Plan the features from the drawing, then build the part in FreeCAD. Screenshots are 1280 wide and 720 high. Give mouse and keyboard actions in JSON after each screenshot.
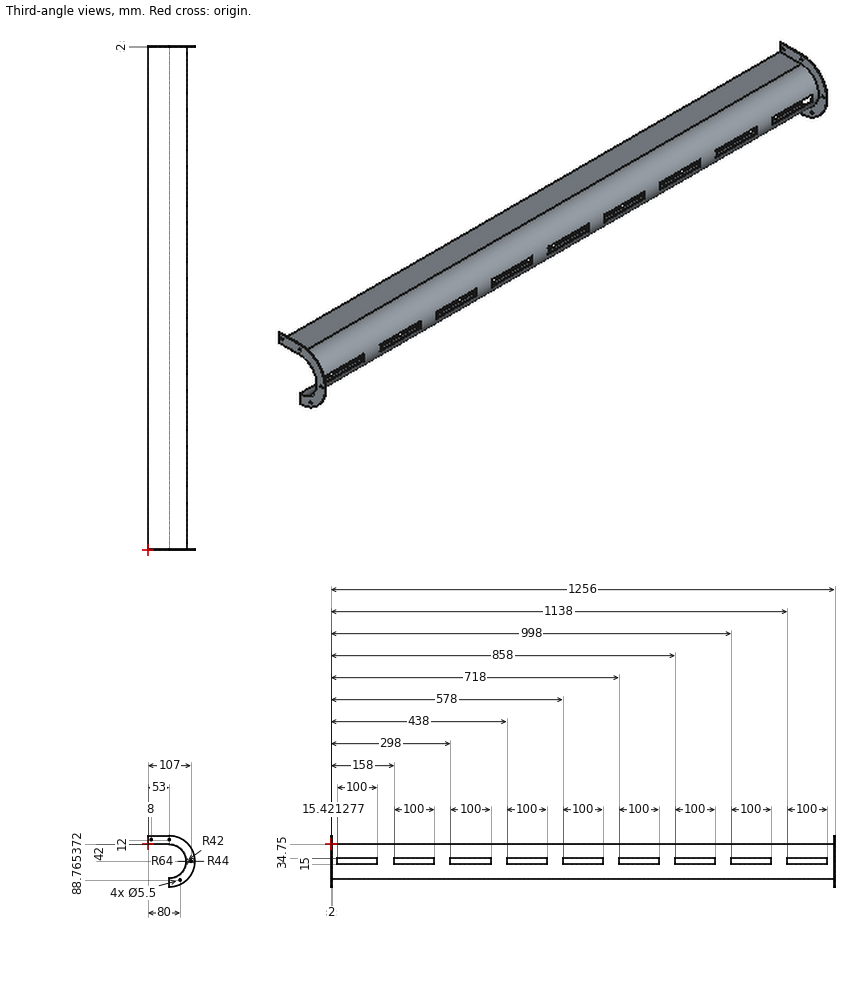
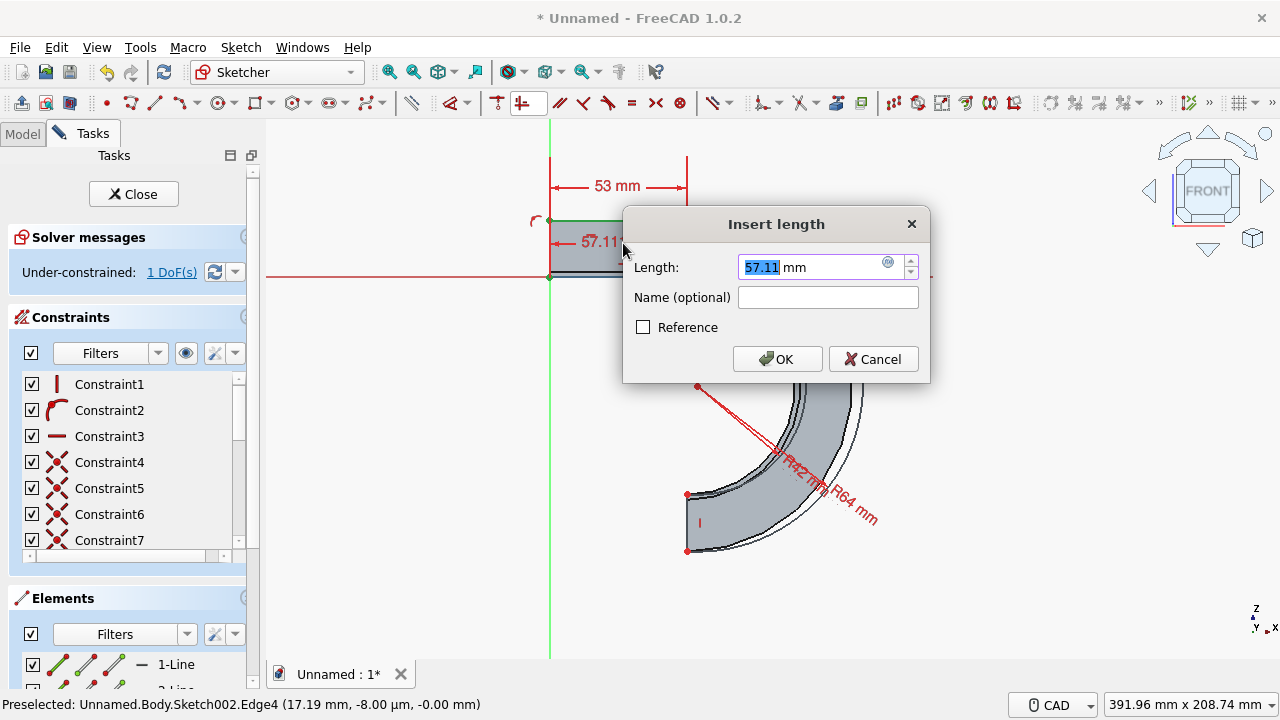
{"action": "type", "text": "53"}
{"action": "key", "text": "Return"}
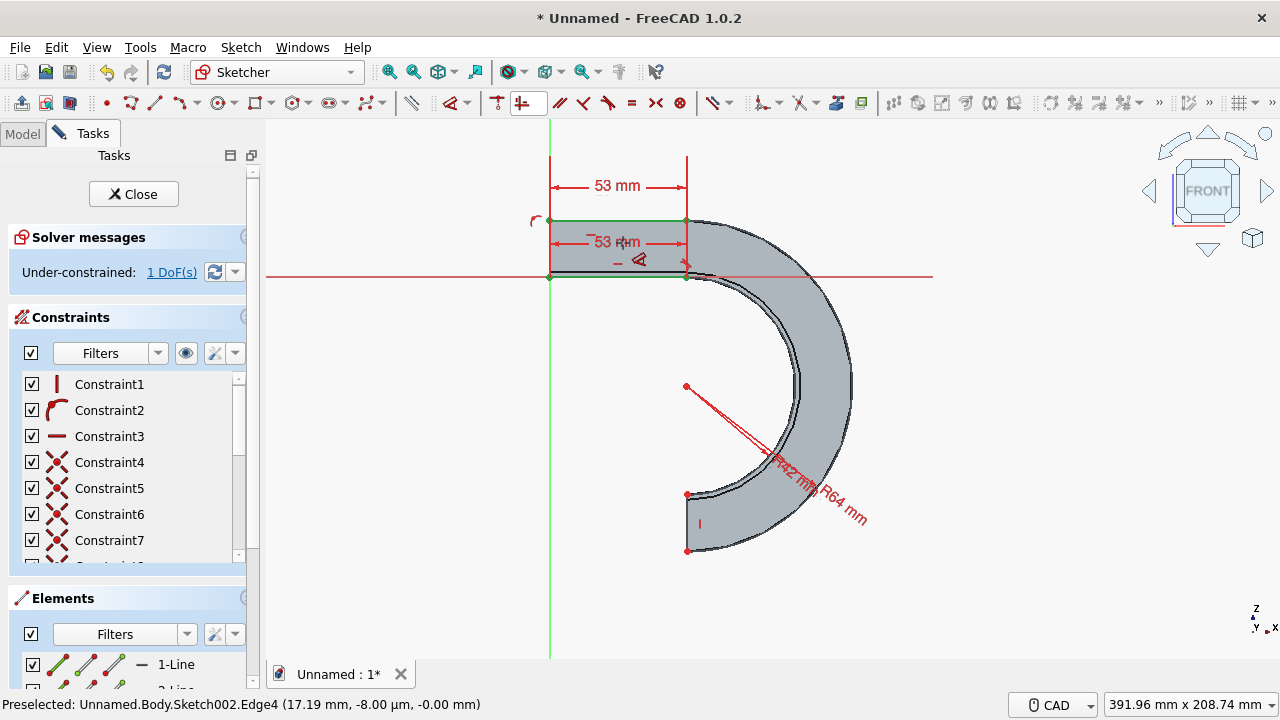
{"action": "left_click", "coordinate": [687, 495]}
{"action": "left_click", "coordinate": [618, 529]}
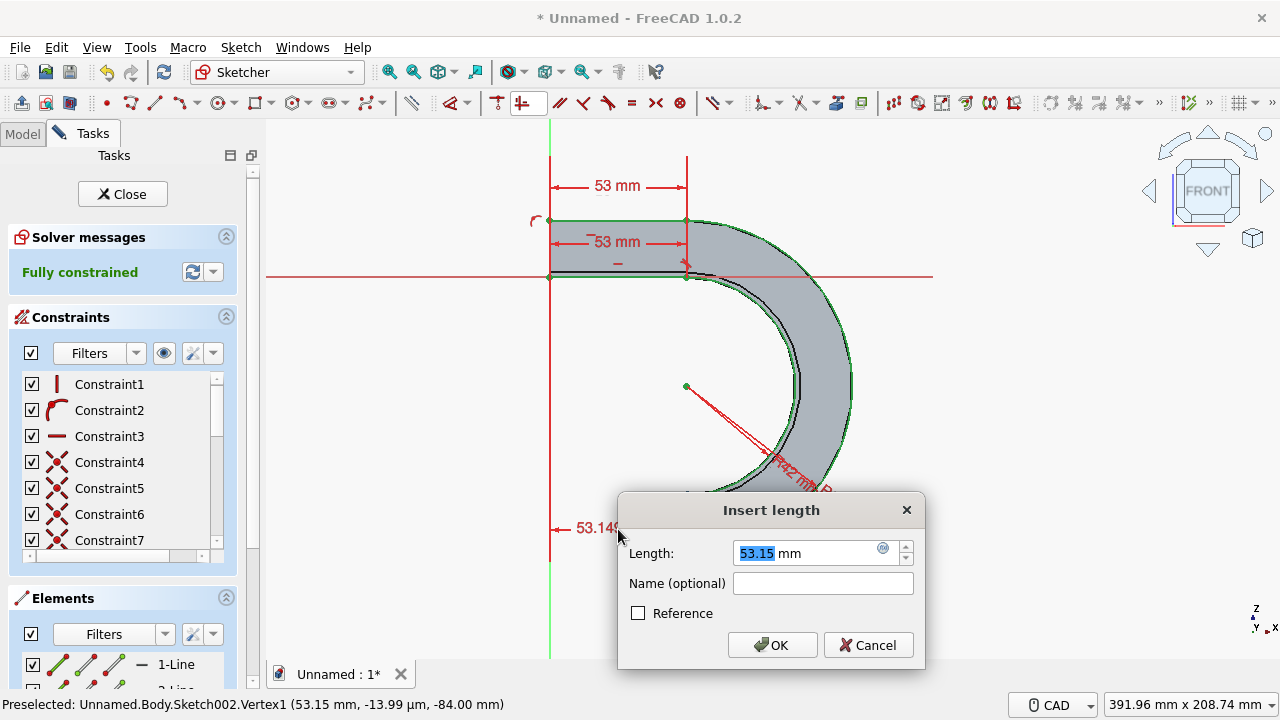
{"action": "type", "text": "53"}
{"action": "key", "text": "Return"}
{"action": "key", "text": "Escape"}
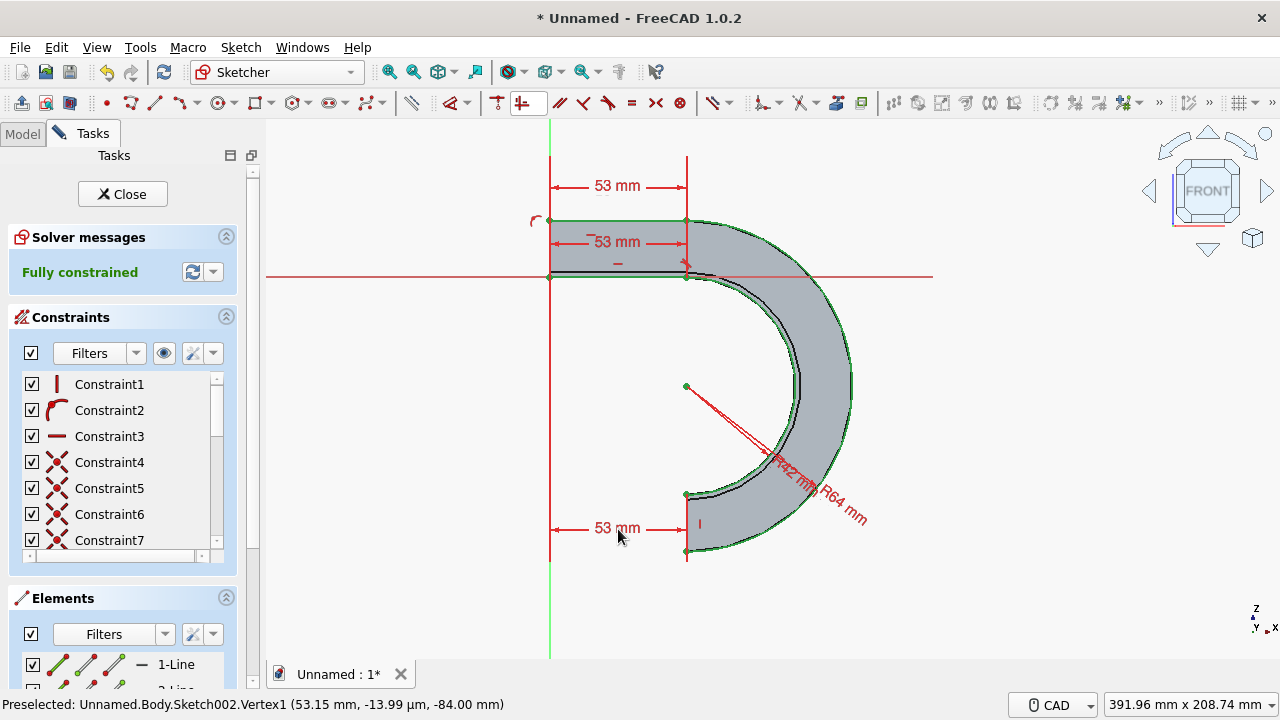
{"action": "left_click", "coordinate": [123, 194]}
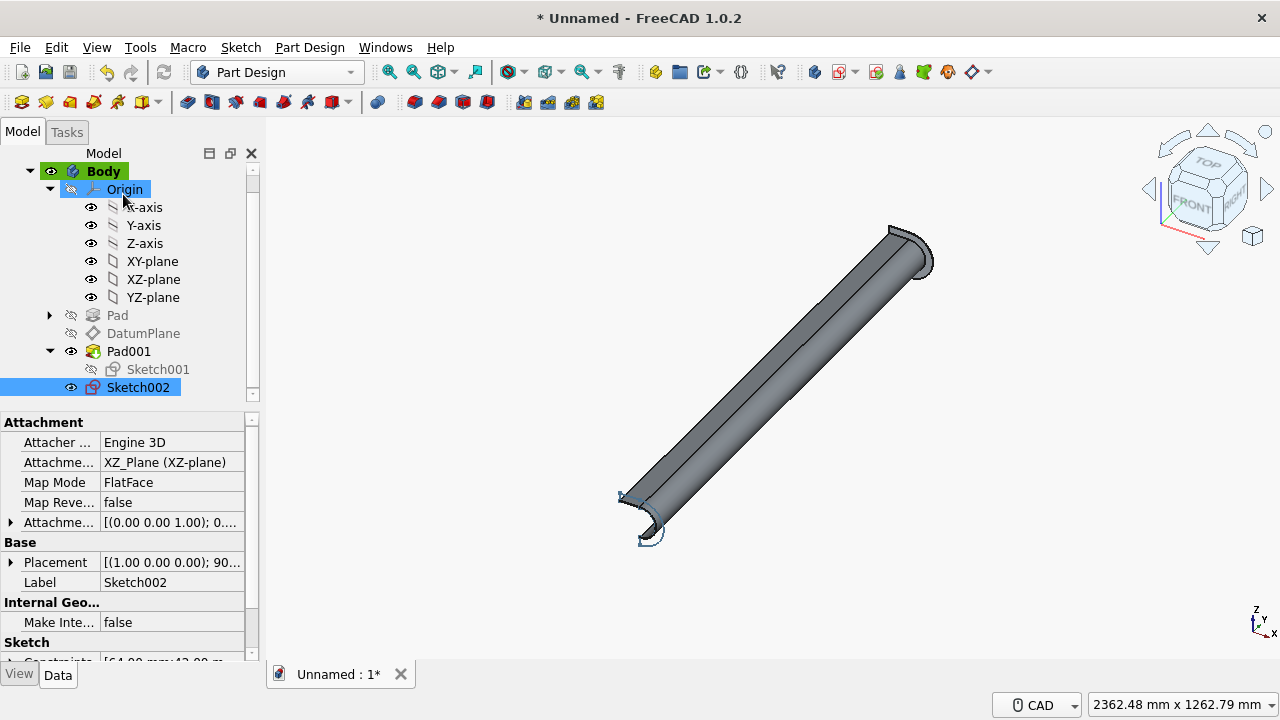
{"action": "left_click", "coordinate": [22, 102]}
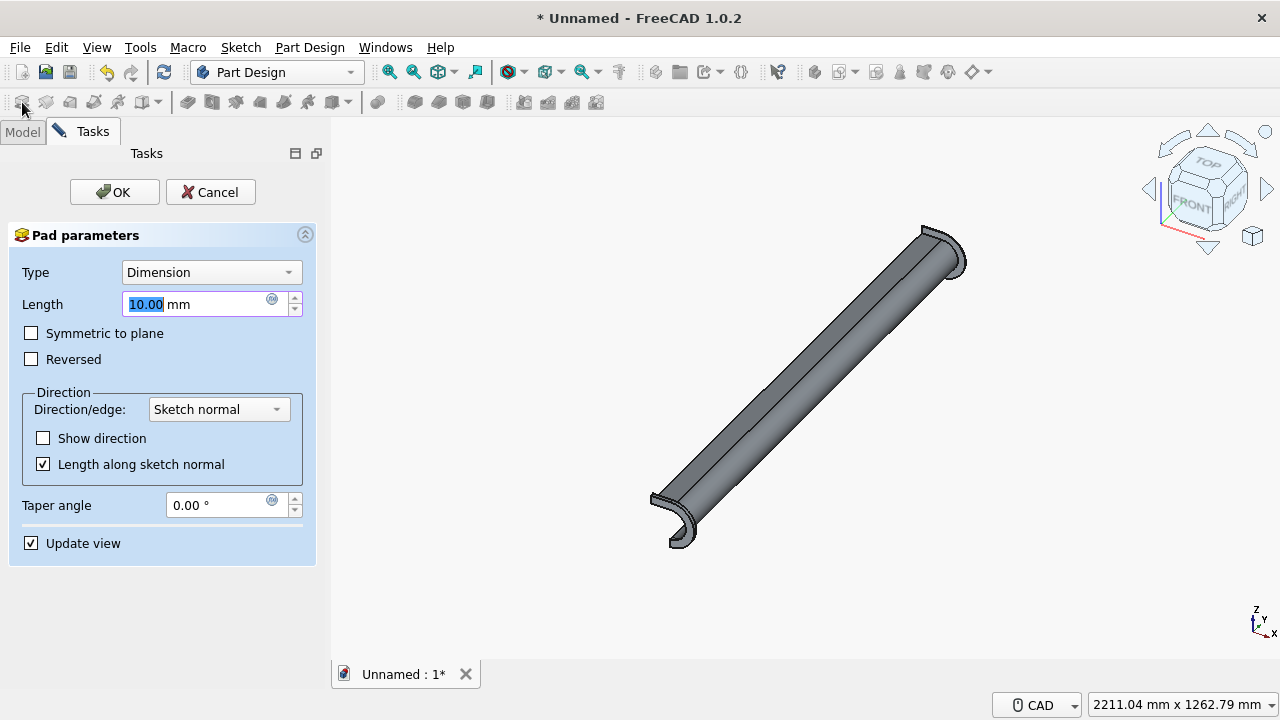
{"action": "type", "text": "2"}
{"action": "key", "text": "Tab"}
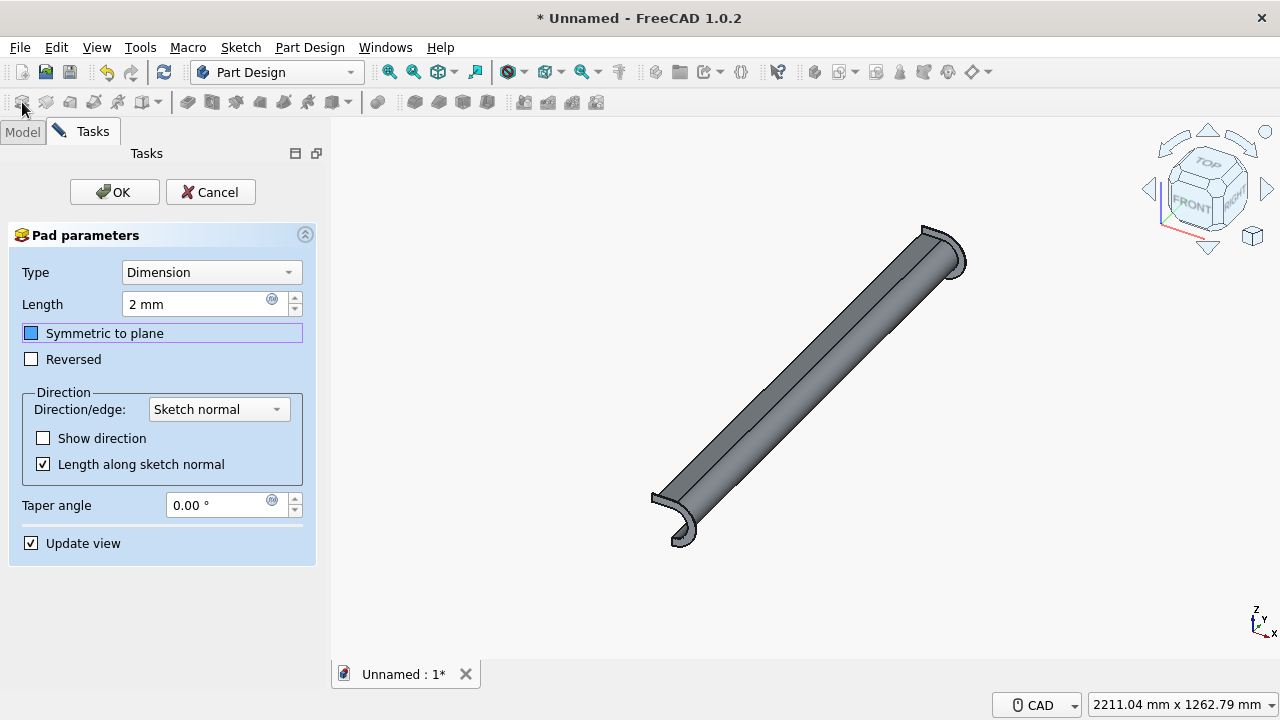
{"action": "left_click", "coordinate": [30, 359]}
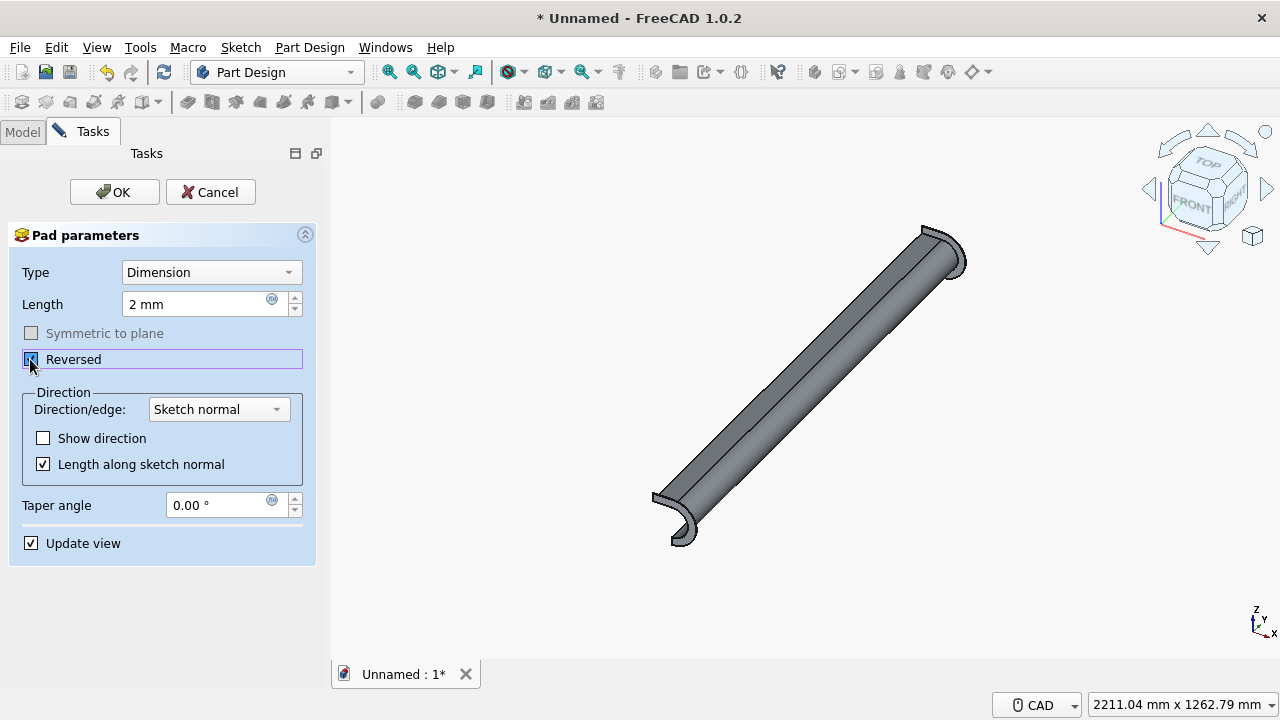
{"action": "left_click", "coordinate": [115, 192]}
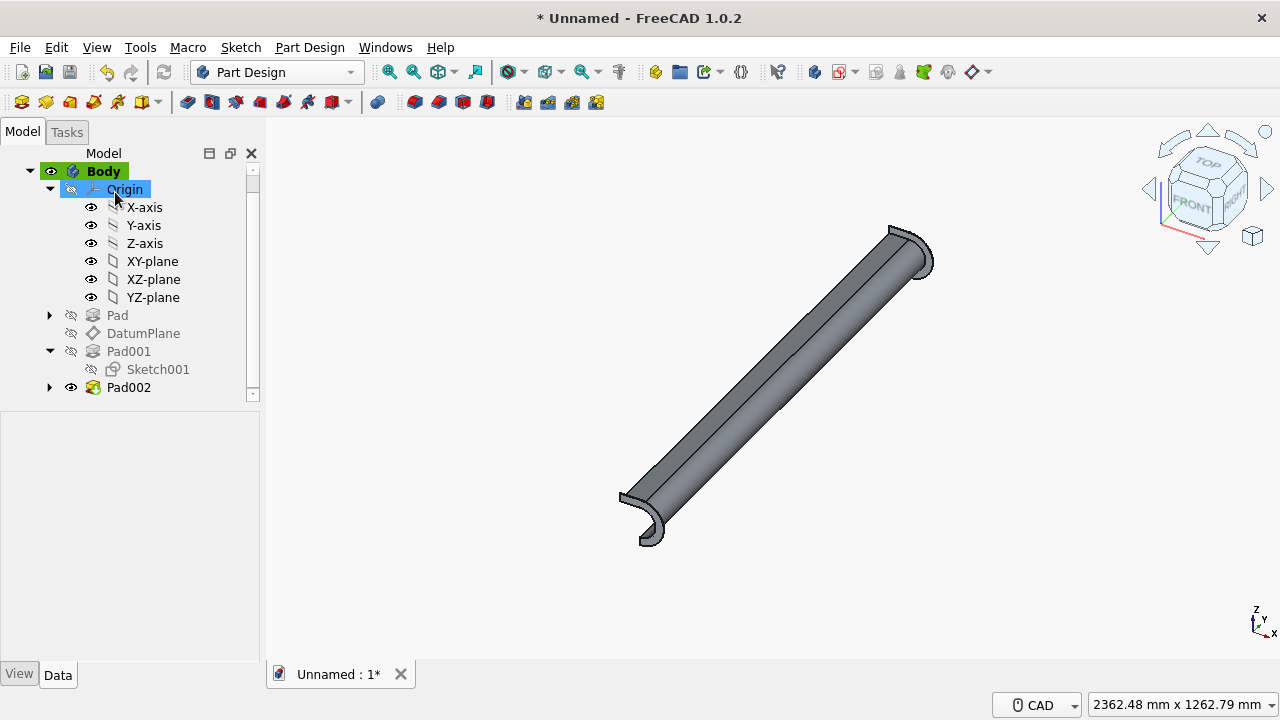
{"action": "key", "text": "6"}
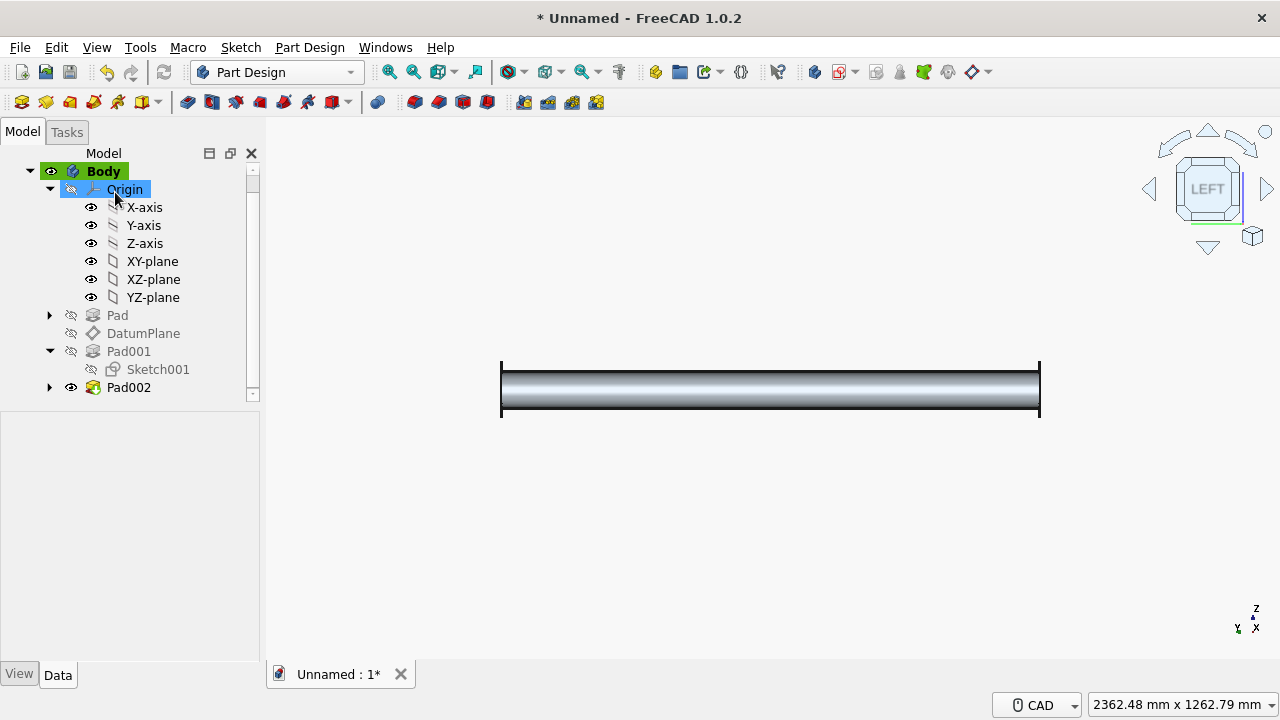
{"action": "scroll", "coordinate": [1002, 370], "scroll_direction": "up", "scroll_amount": 15}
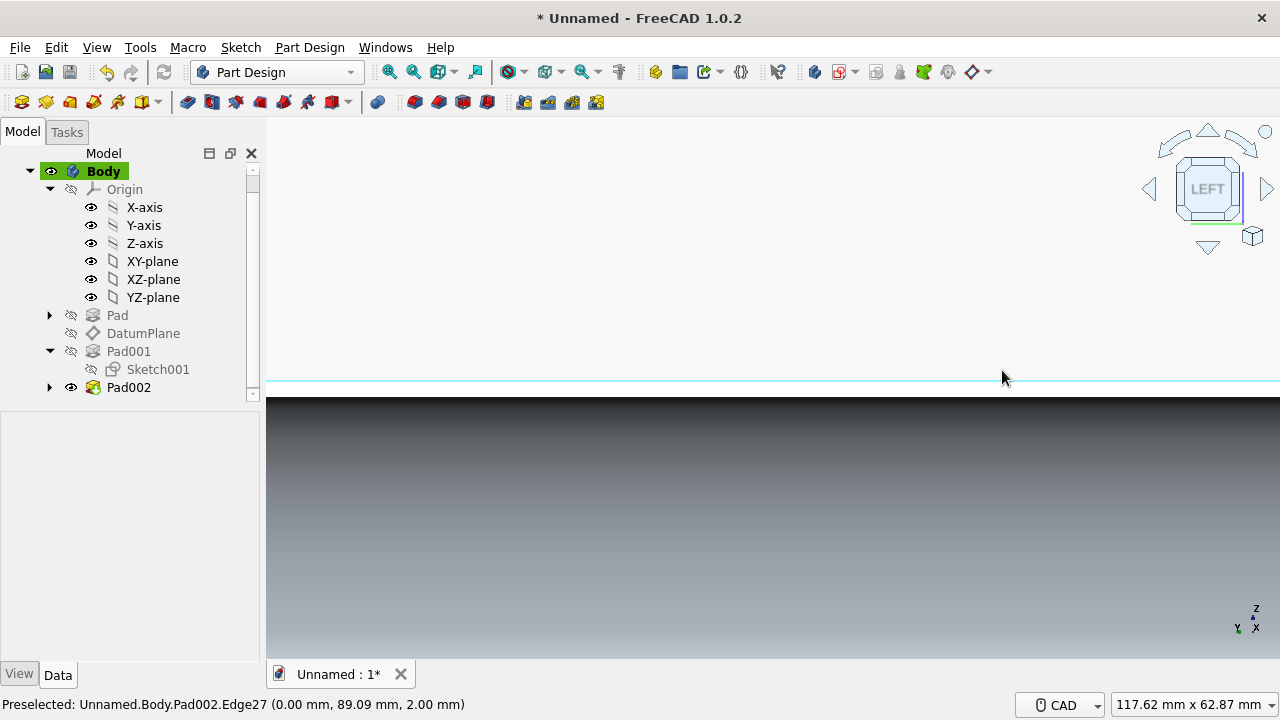
{"action": "scroll", "coordinate": [983, 384], "scroll_direction": "up", "scroll_amount": 6}